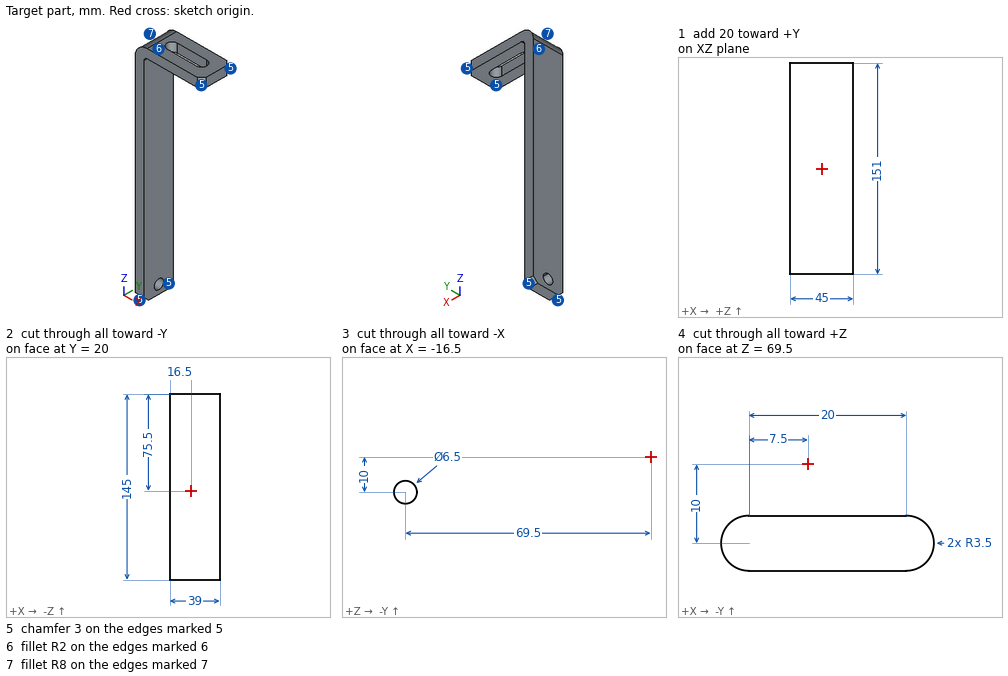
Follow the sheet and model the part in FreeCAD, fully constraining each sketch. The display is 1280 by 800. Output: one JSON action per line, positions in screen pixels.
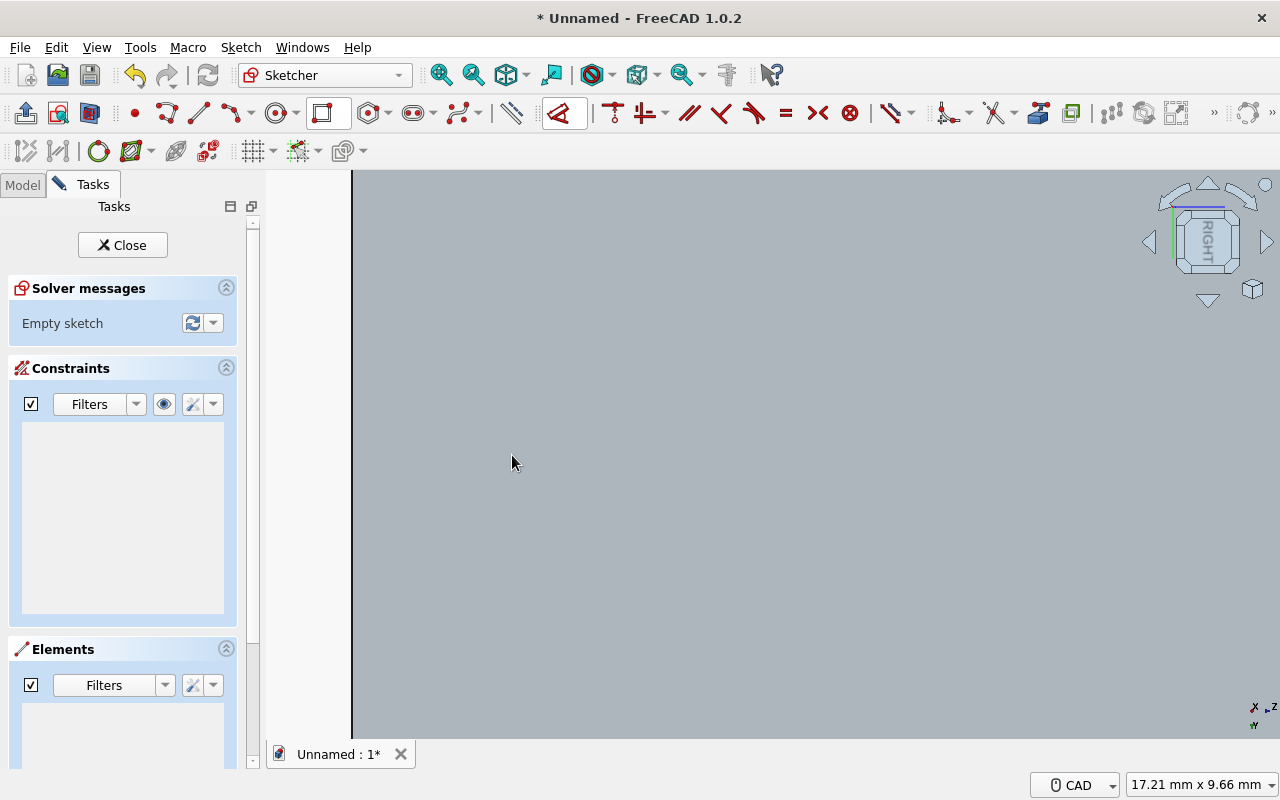
{"action": "left_click", "coordinate": [276, 114]}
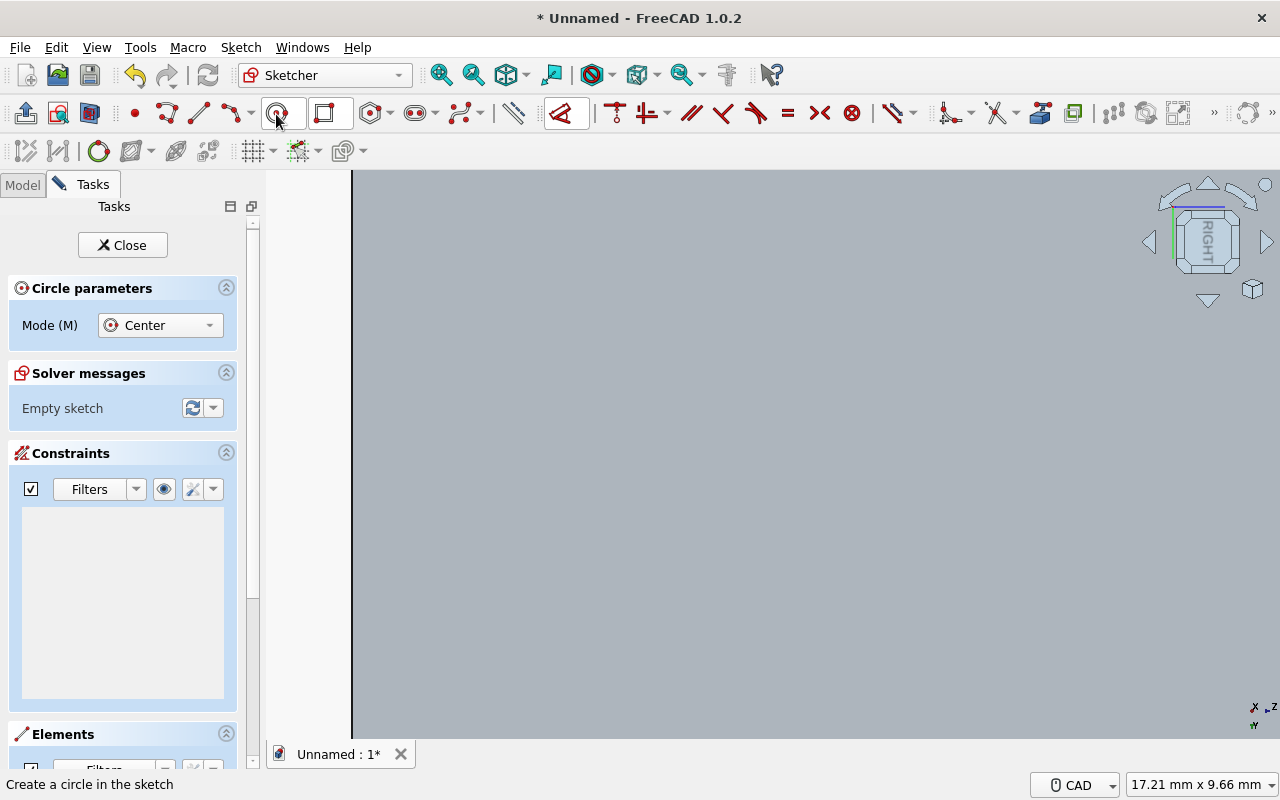
{"action": "left_click", "coordinate": [706, 439]}
{"action": "left_click", "coordinate": [841, 304]}
{"action": "key", "text": "Escape"}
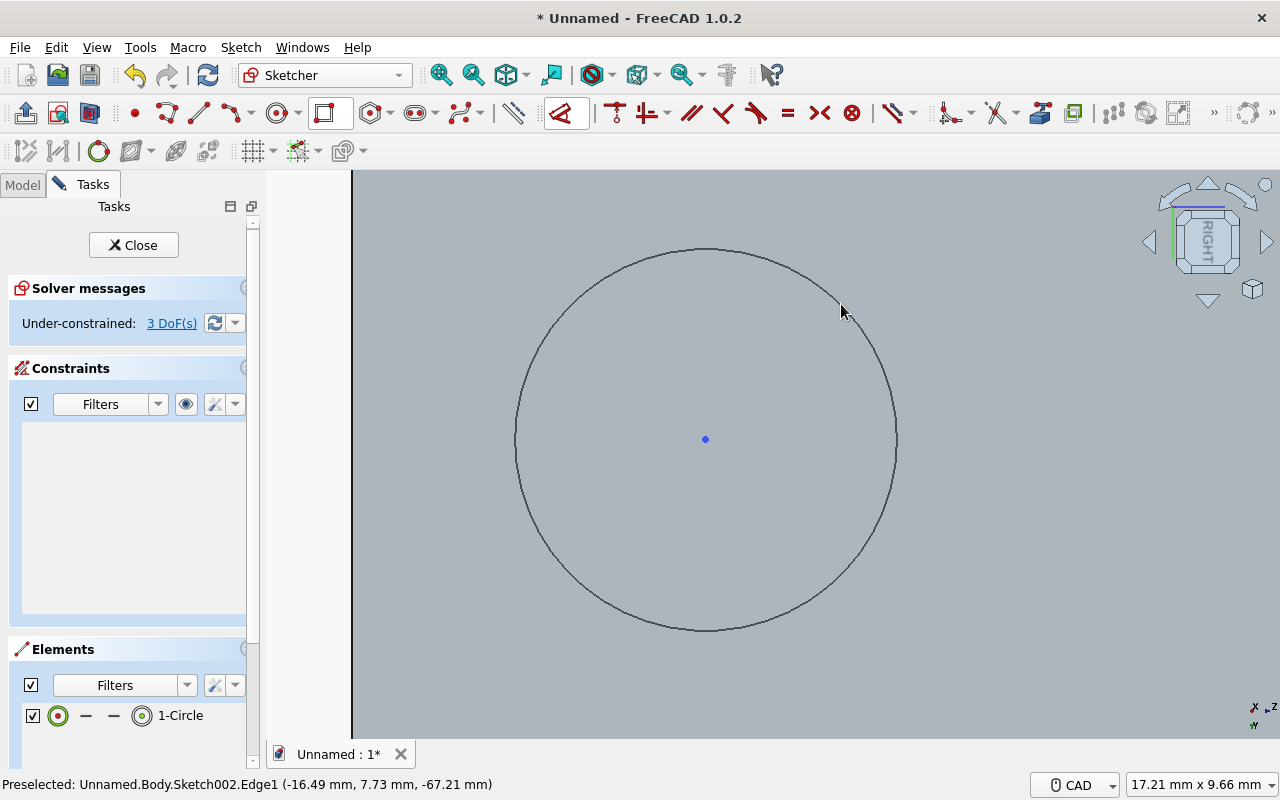
{"action": "left_click", "coordinate": [841, 305]}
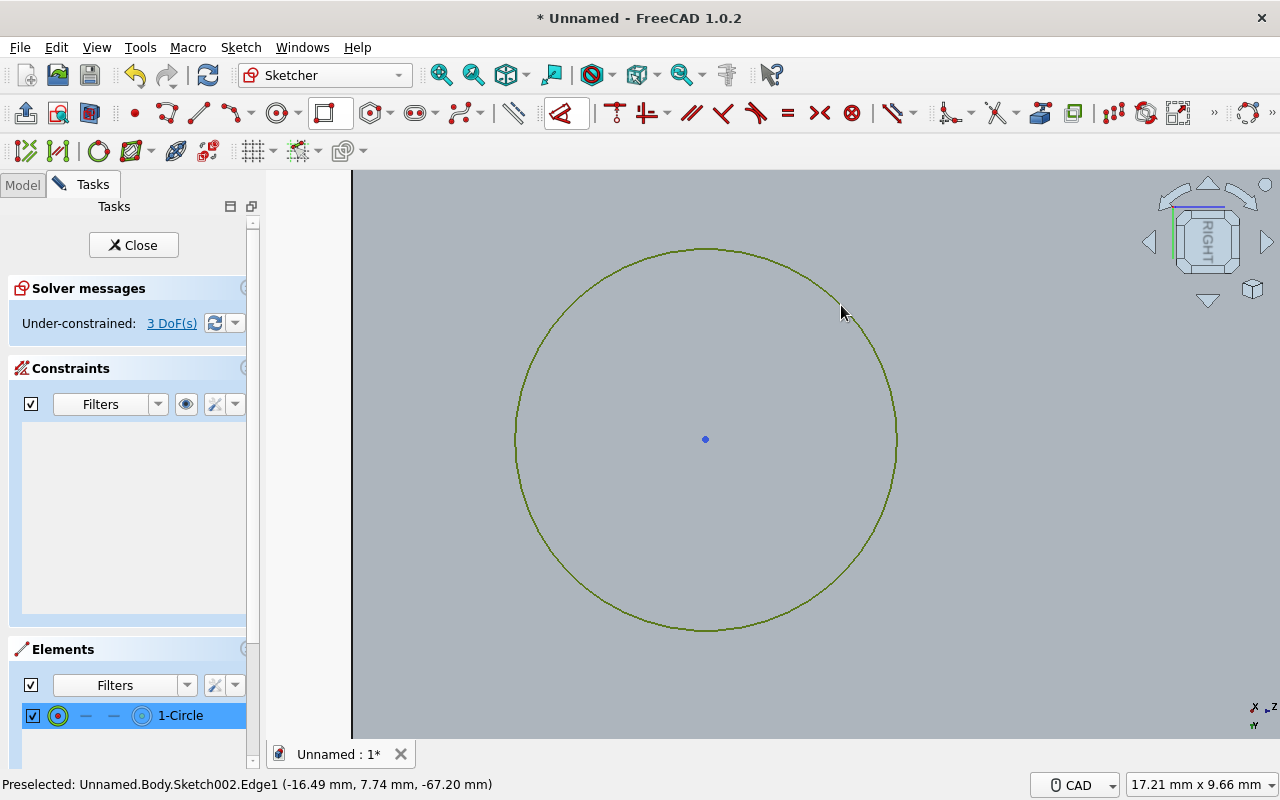
{"action": "left_click", "coordinate": [584, 114]}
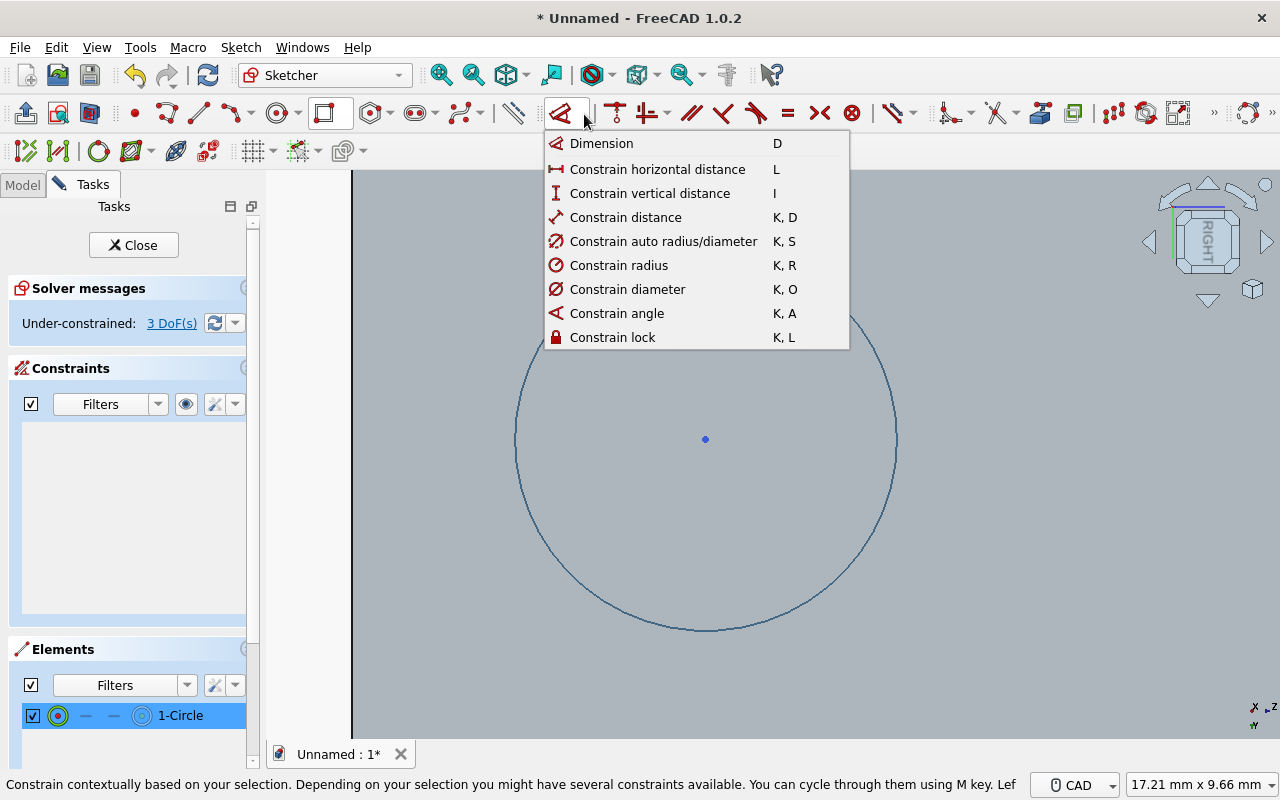
{"action": "left_click", "coordinate": [697, 289]}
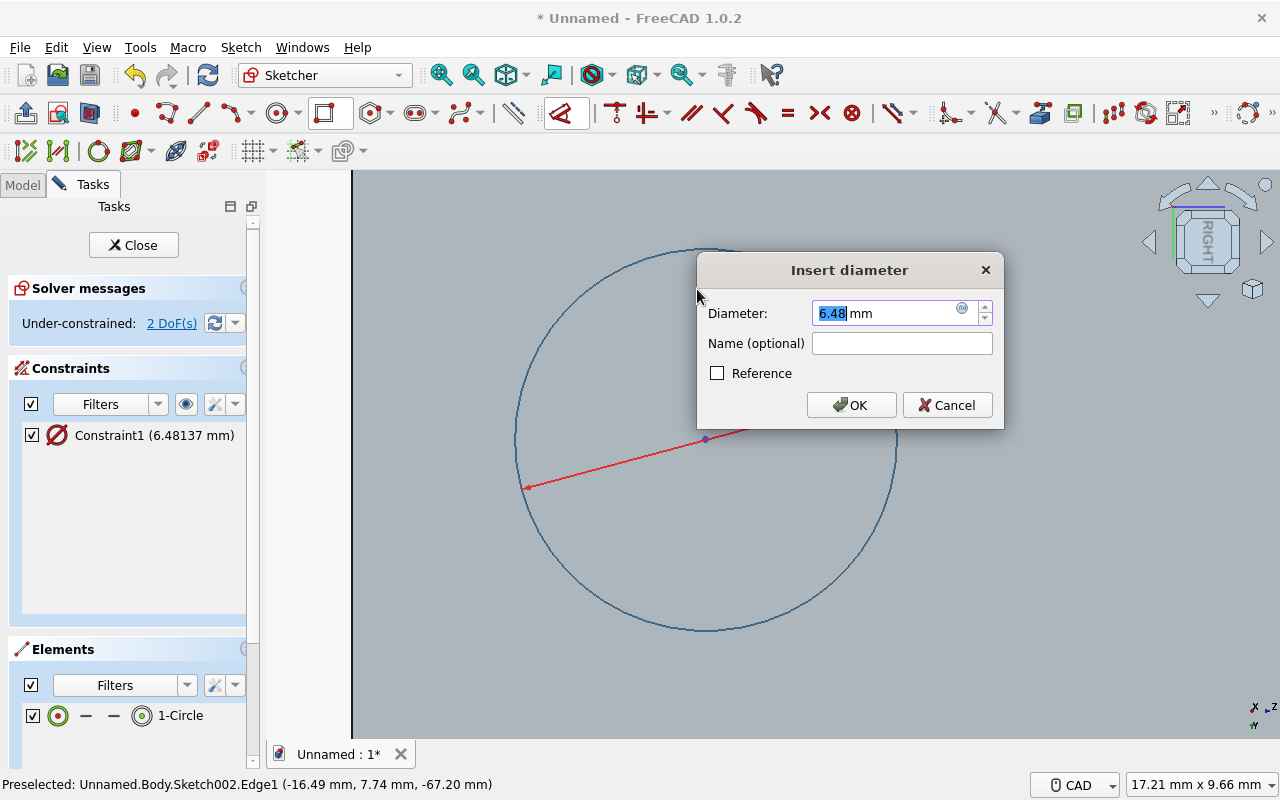
{"action": "type", "text": "6.5"}
{"action": "key", "text": "Return"}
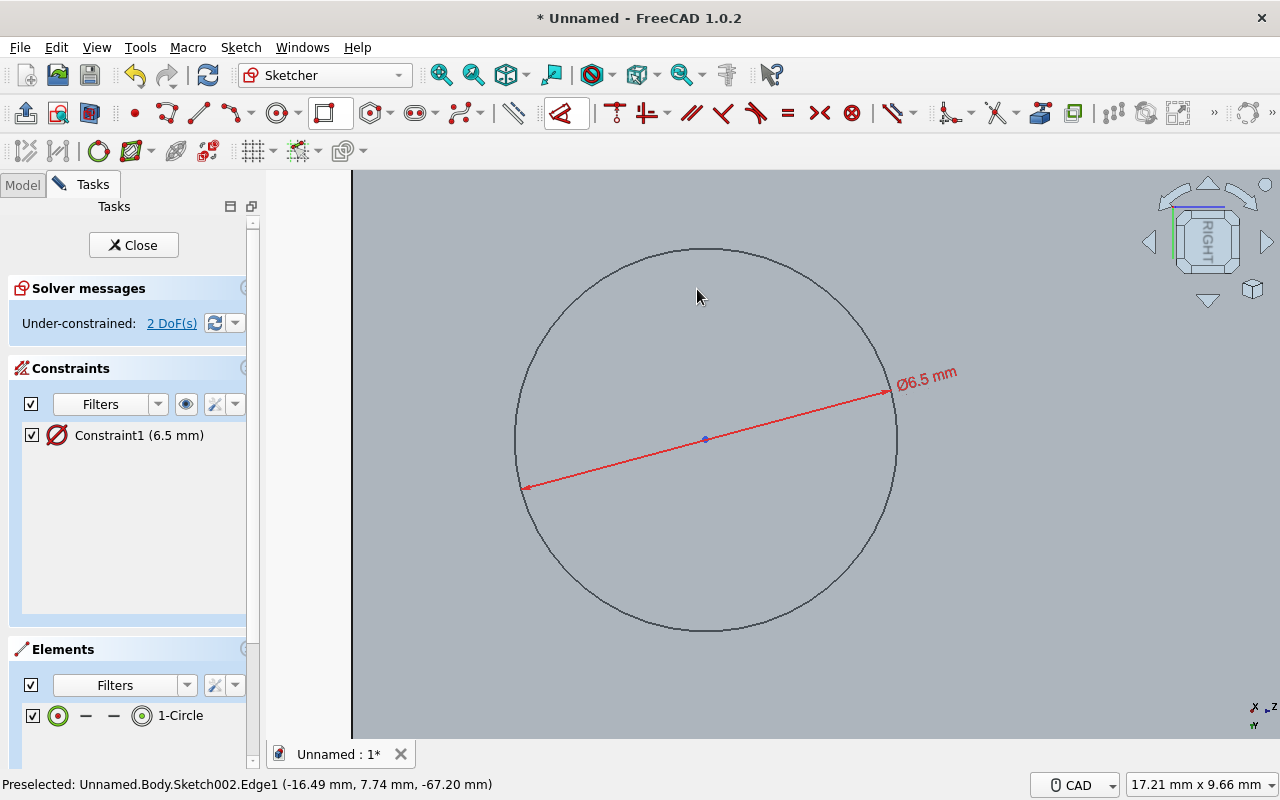
{"action": "left_click", "coordinate": [706, 440]}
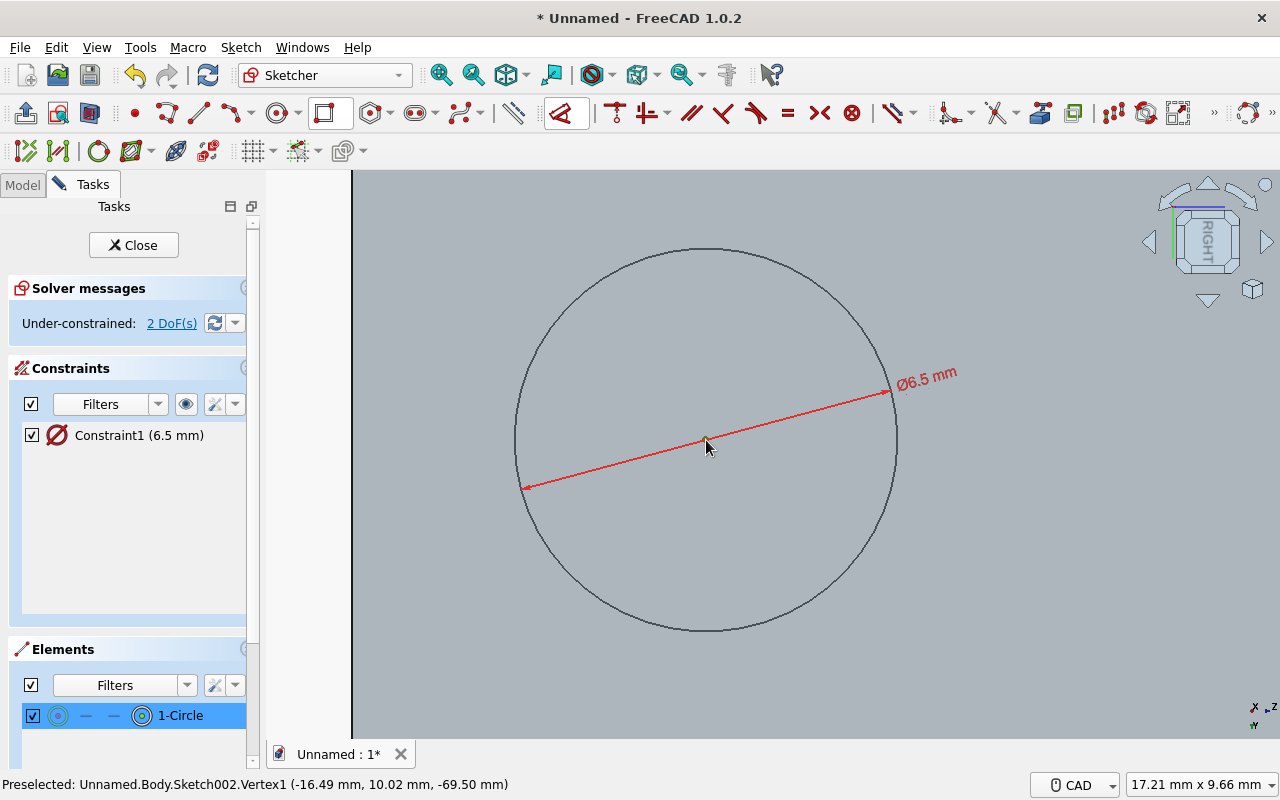
{"action": "left_click", "coordinate": [584, 114]}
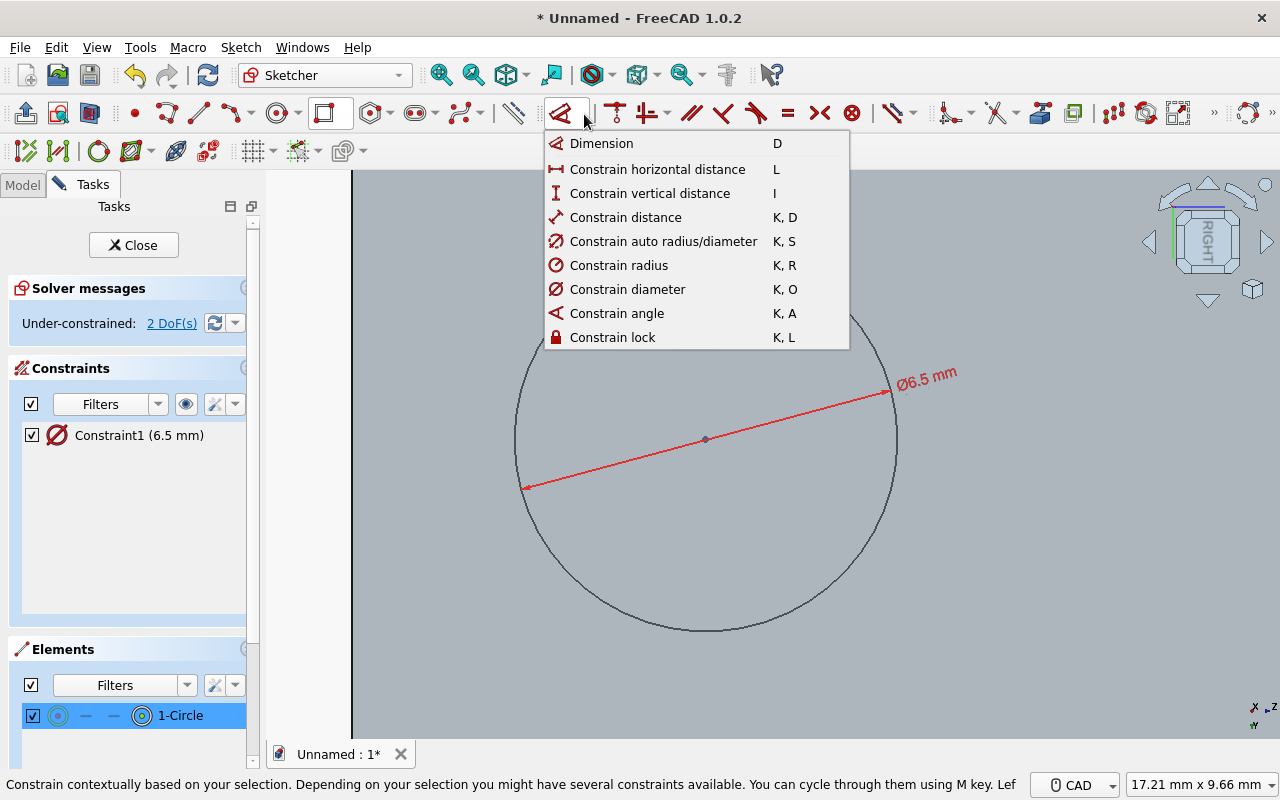
{"action": "left_click", "coordinate": [697, 193]}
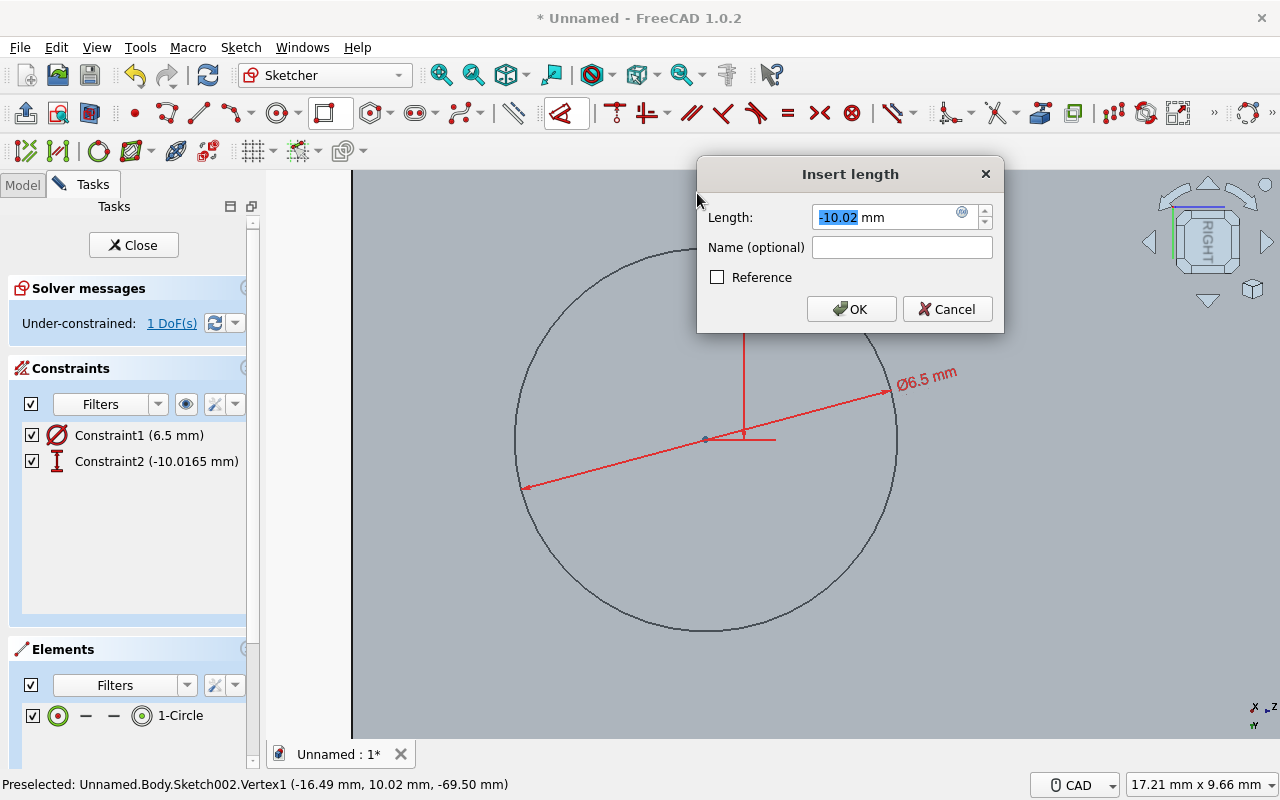
{"action": "type", "text": "-10"}
{"action": "key", "text": "Return"}